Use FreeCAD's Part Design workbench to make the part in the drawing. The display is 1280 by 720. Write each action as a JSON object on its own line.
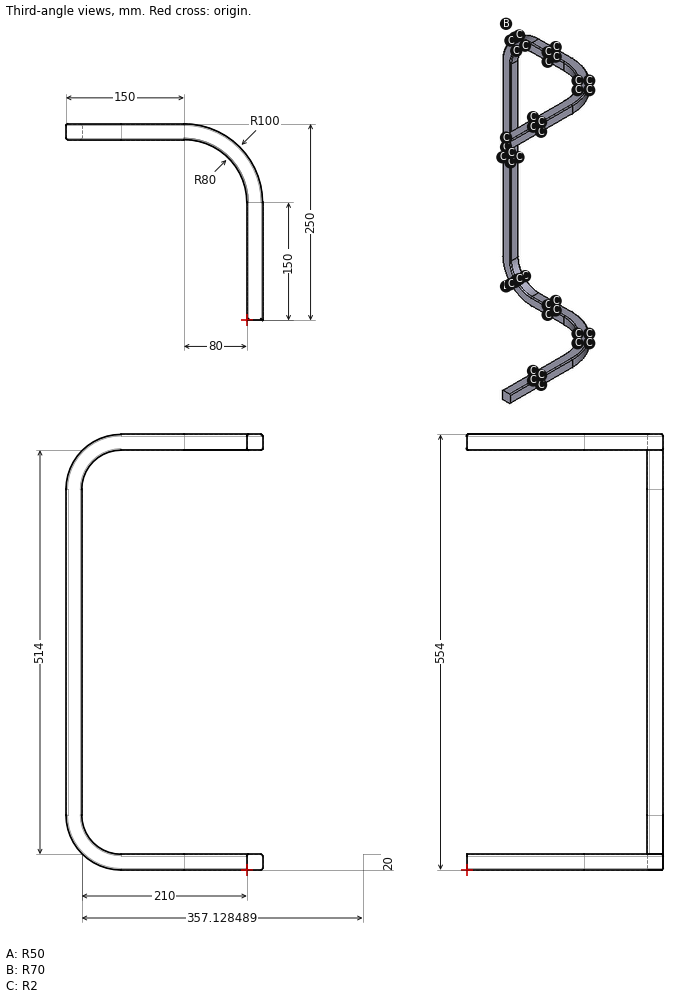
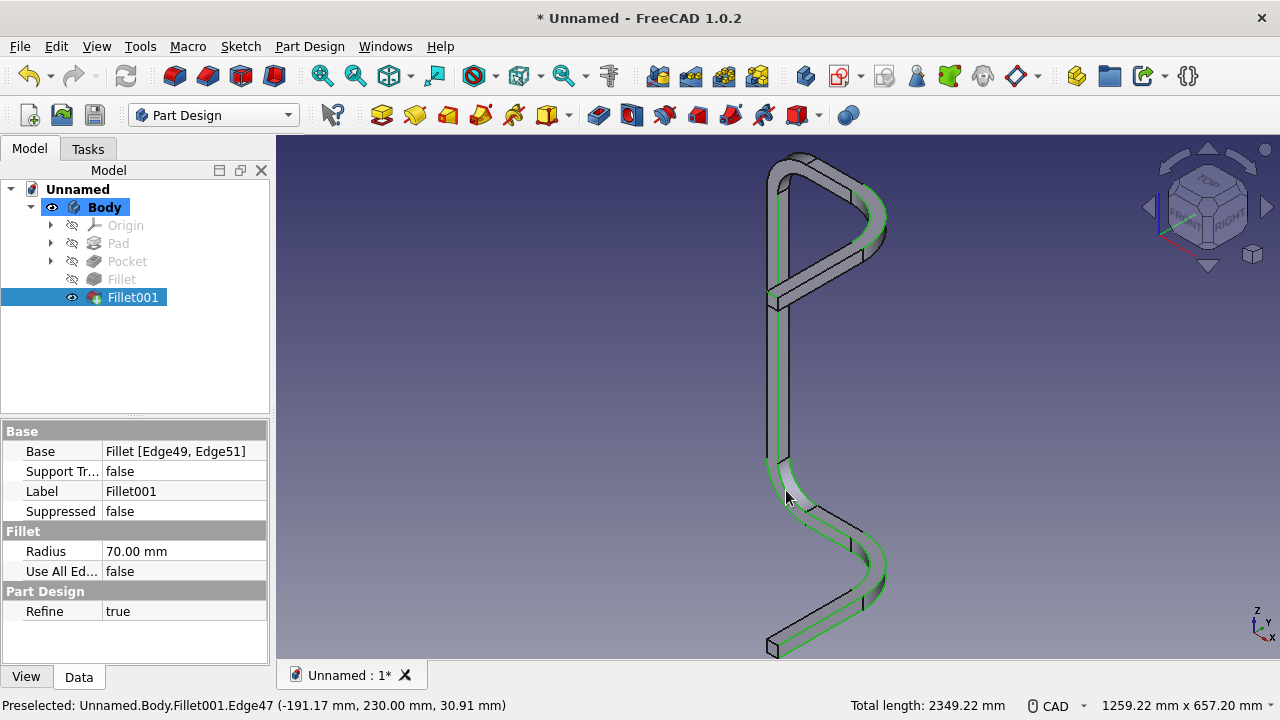
{"action": "left_click", "coordinate": [783, 177], "text": "ctrl"}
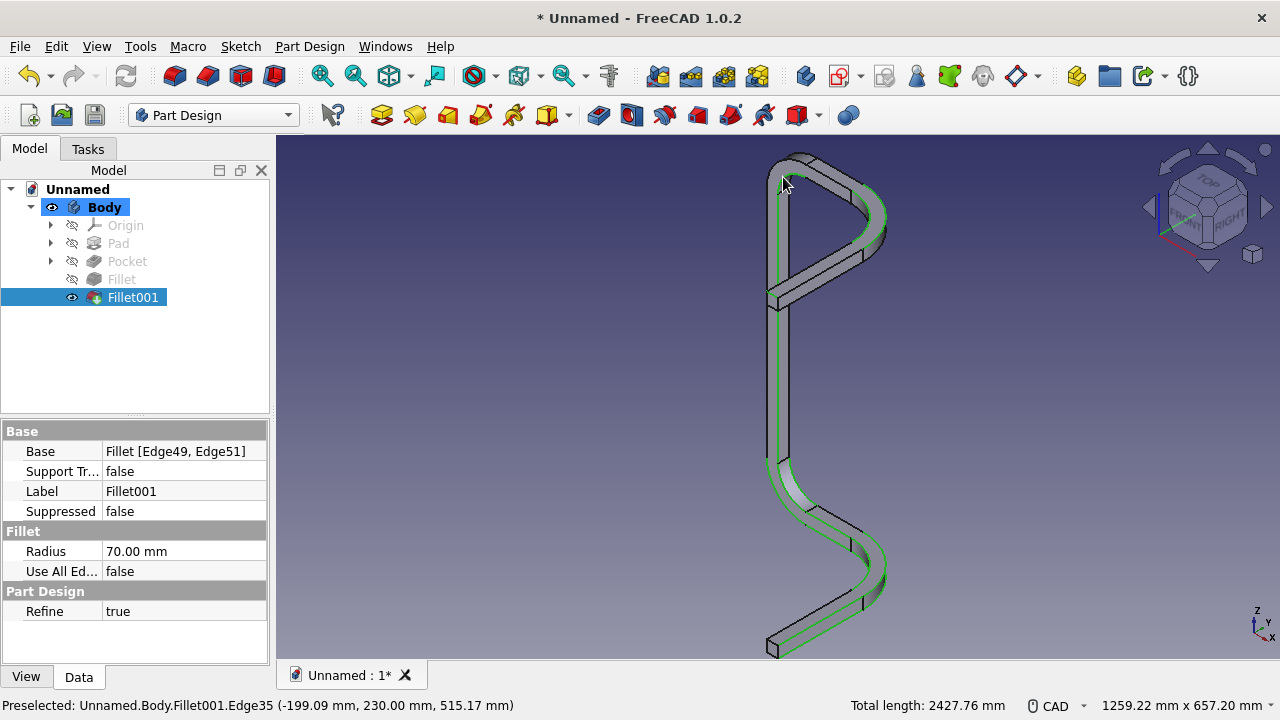
{"action": "left_click", "coordinate": [820, 273], "text": "ctrl"}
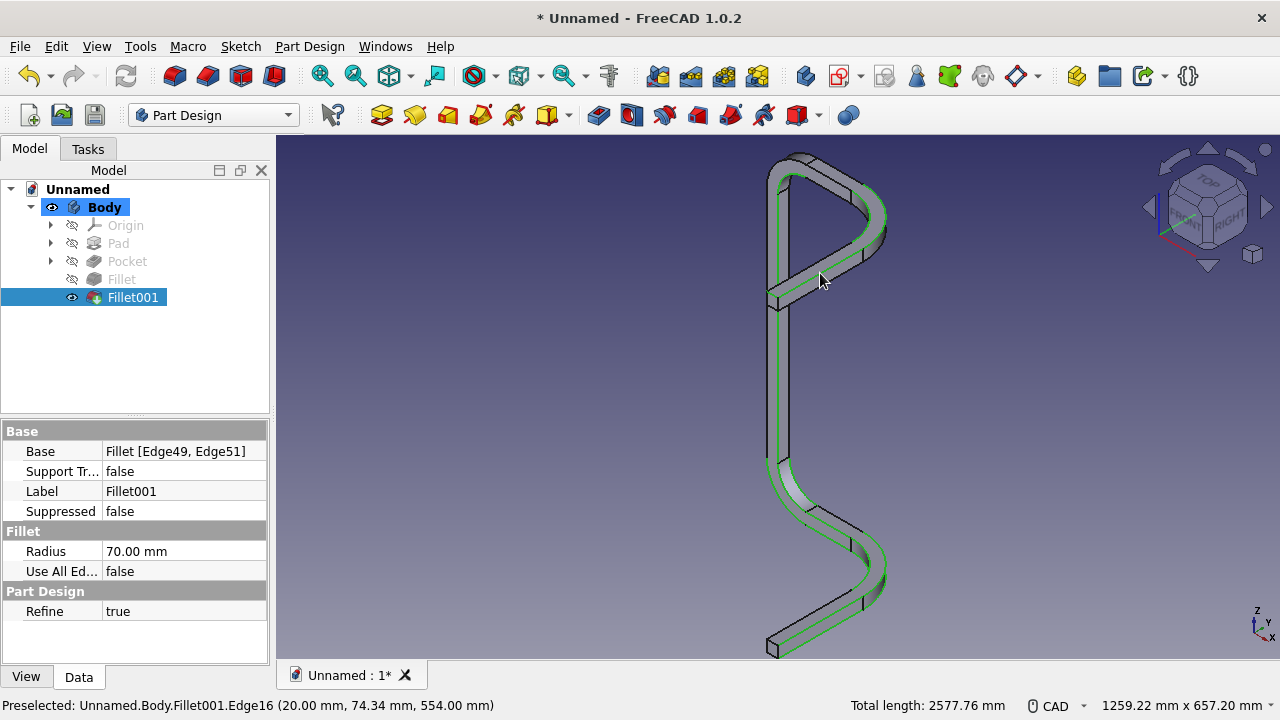
{"action": "left_click", "coordinate": [829, 177], "text": "ctrl"}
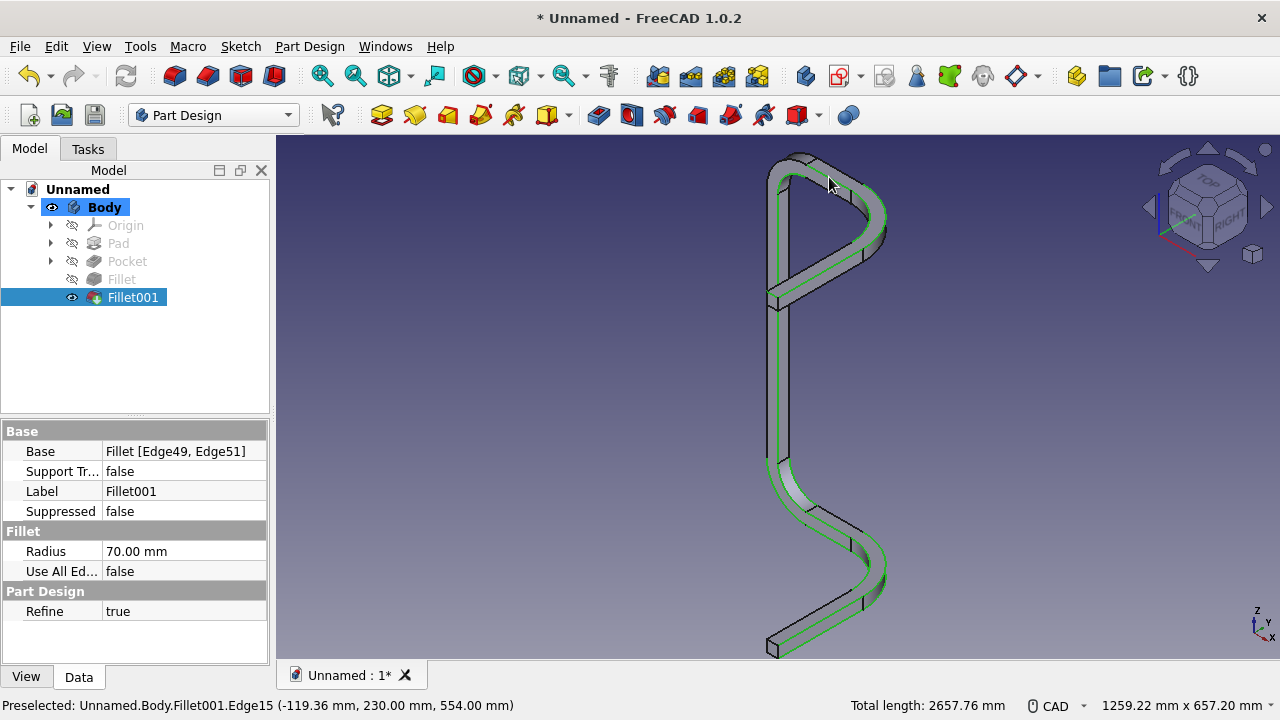
{"action": "left_click", "coordinate": [769, 173], "text": "ctrl"}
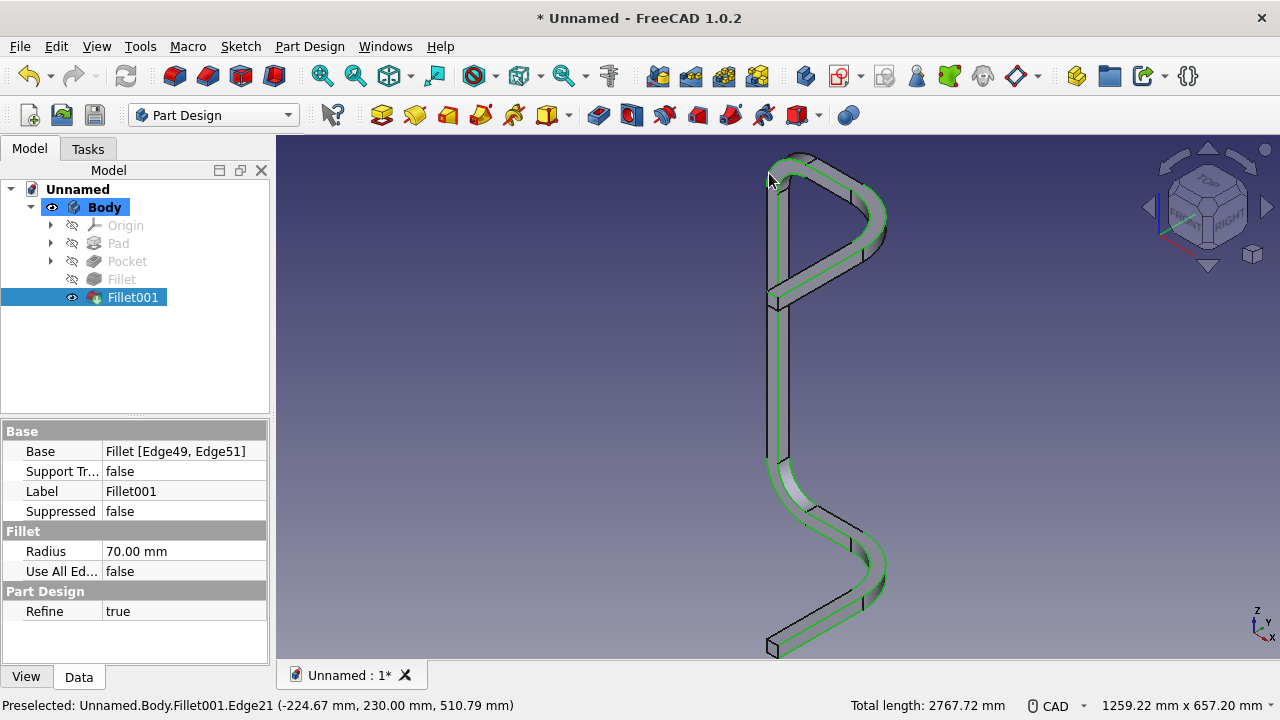
{"action": "key", "text": "2"}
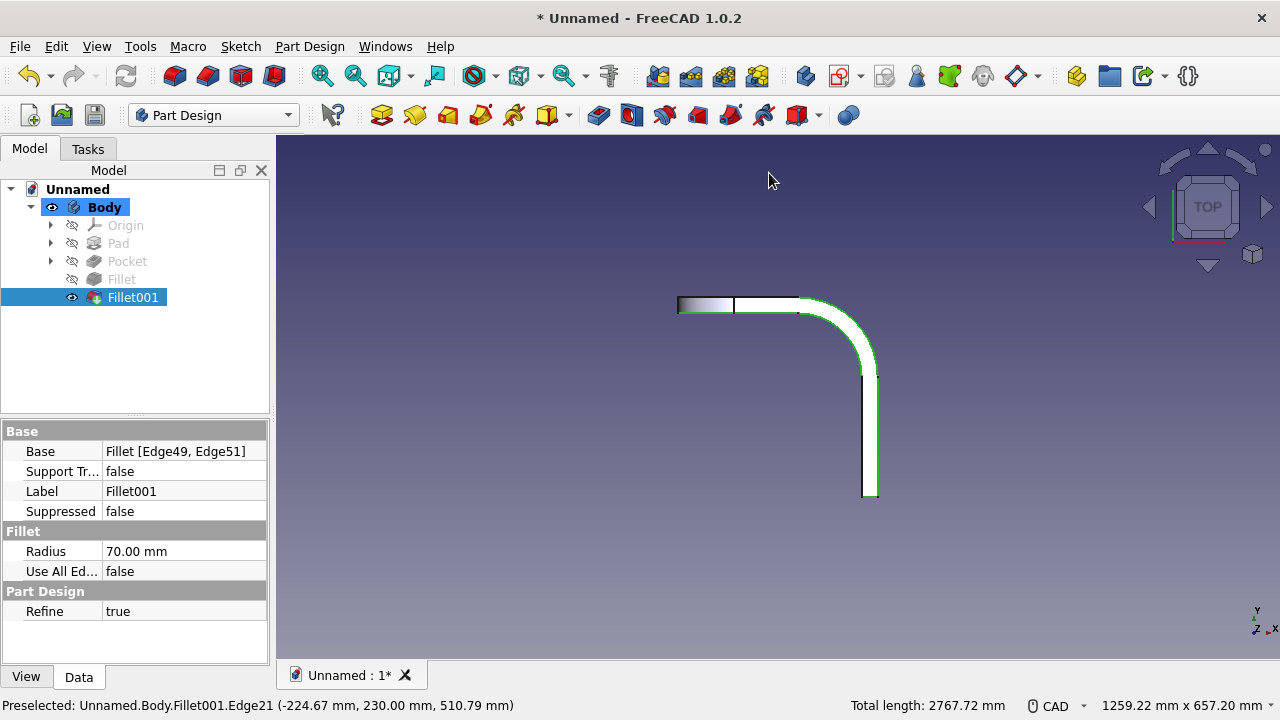
{"action": "left_click", "coordinate": [323, 76]}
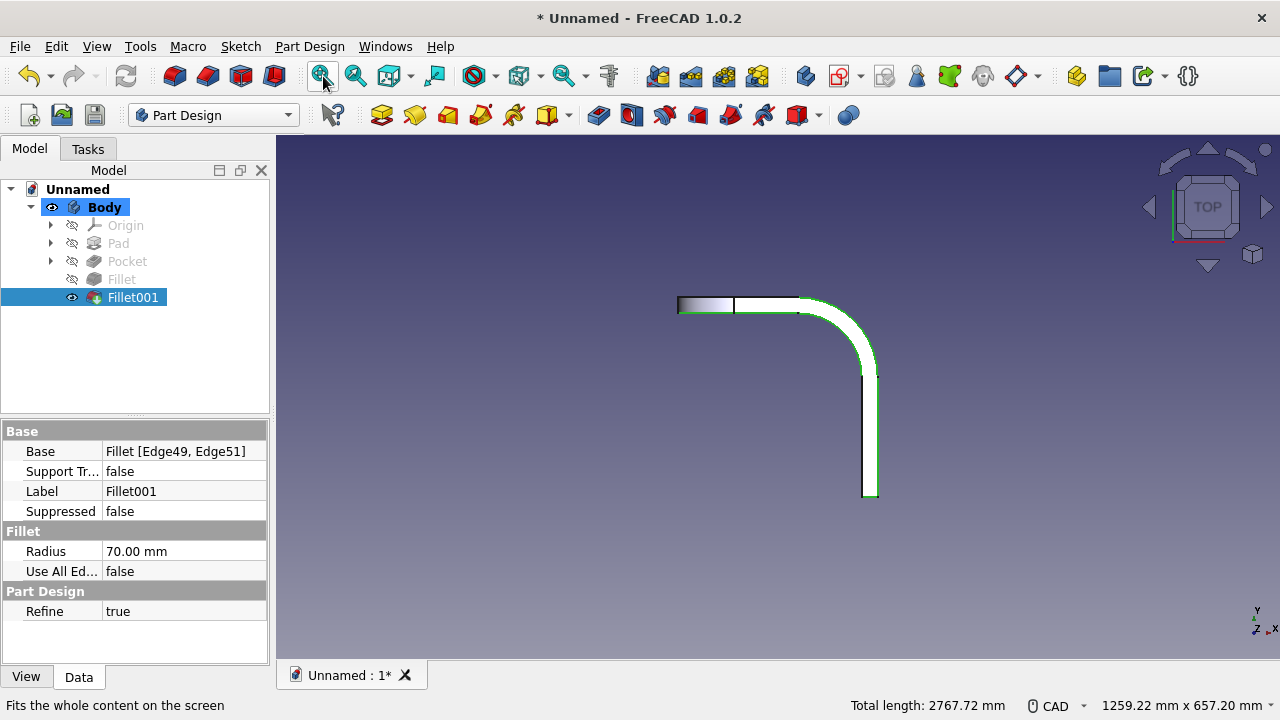
{"action": "left_click", "coordinate": [766, 296], "text": "ctrl"}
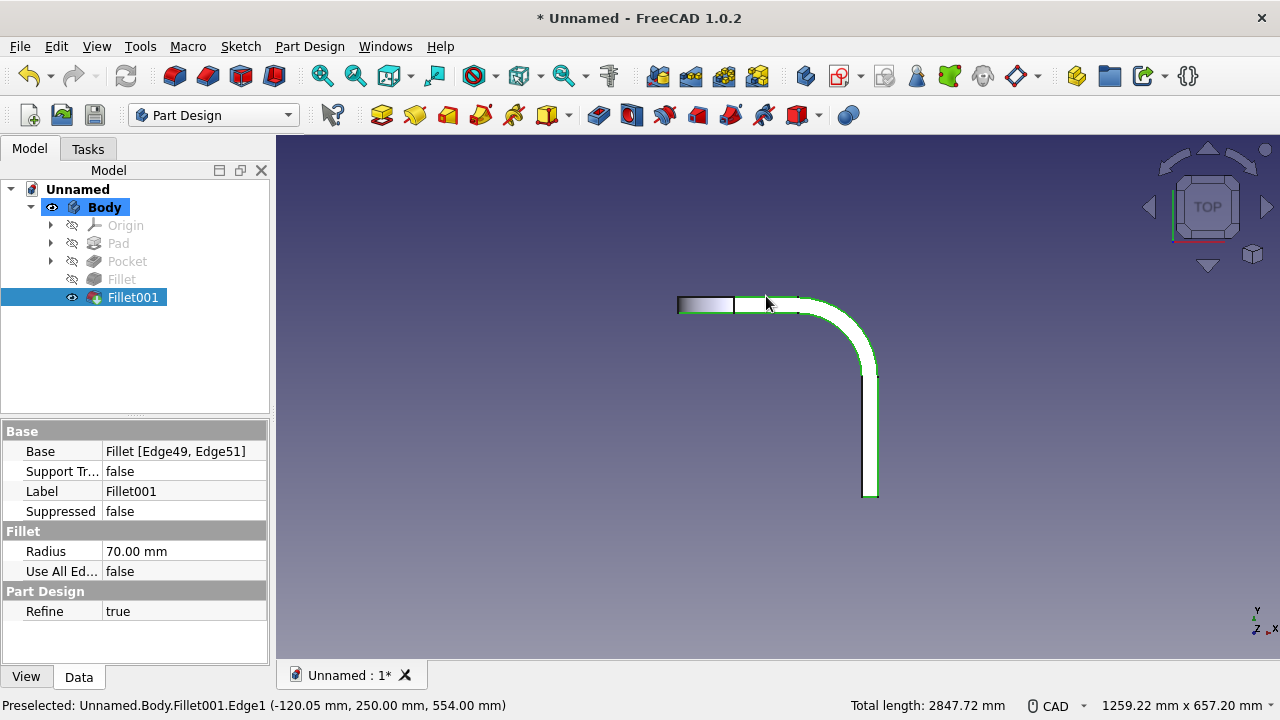
{"action": "left_click", "coordinate": [862, 436], "text": "ctrl"}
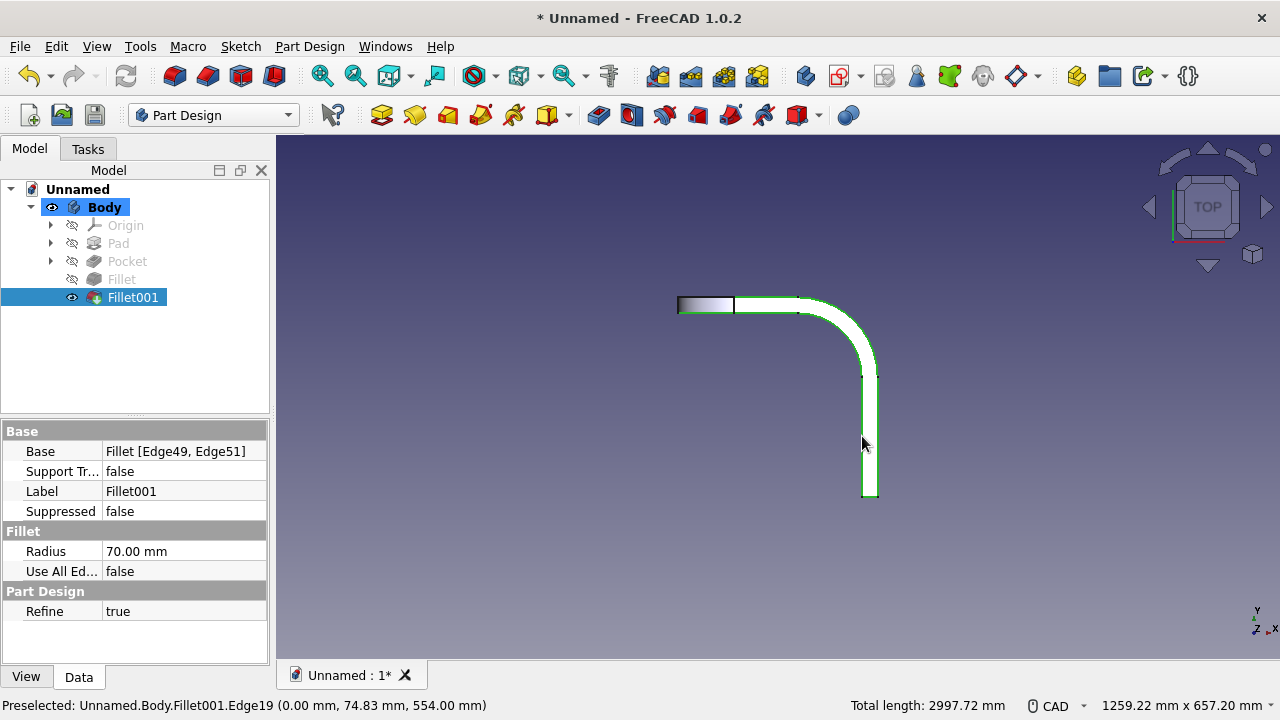
{"action": "left_click", "coordinate": [695, 296], "text": "ctrl"}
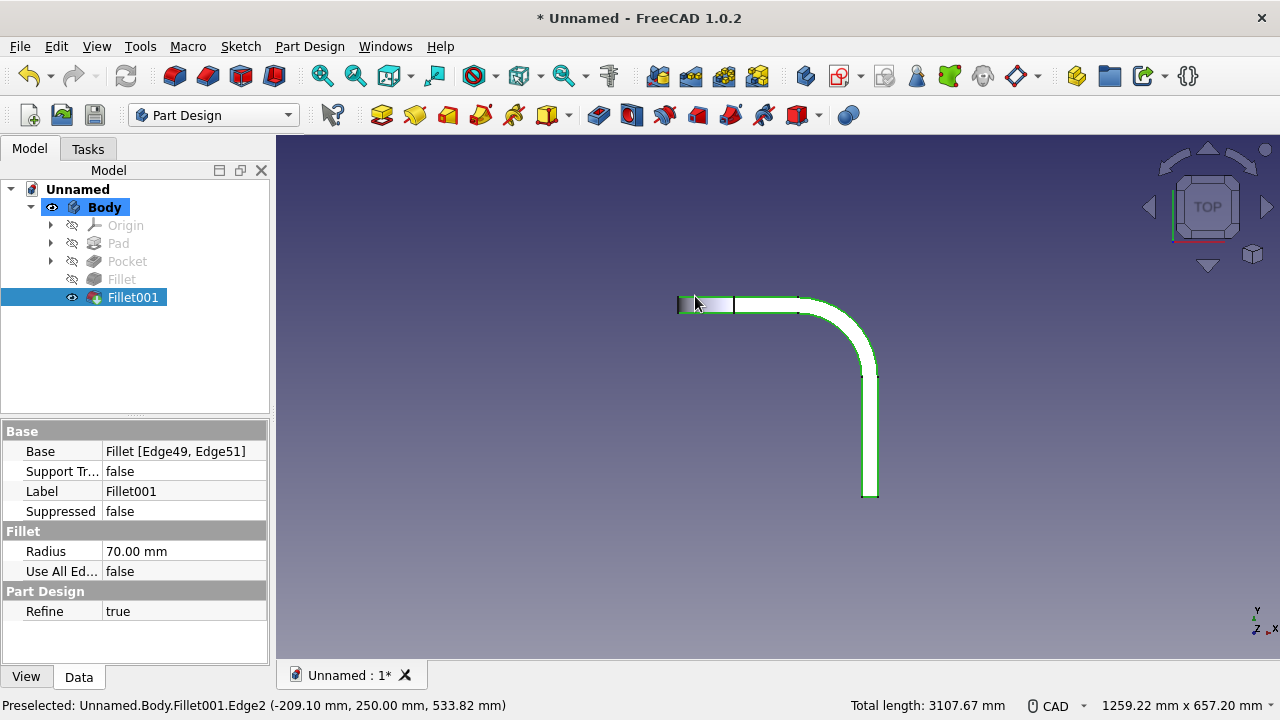
{"action": "key", "text": "1"}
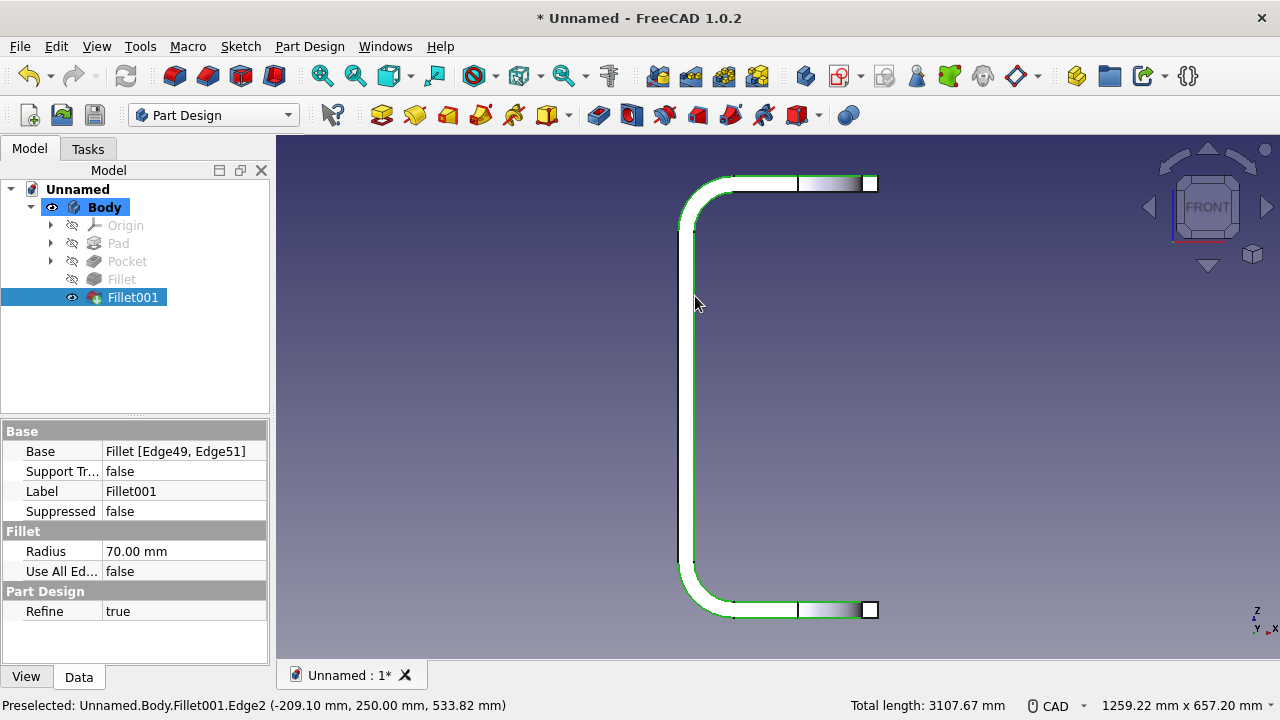
{"action": "left_click", "coordinate": [843, 191], "text": "ctrl"}